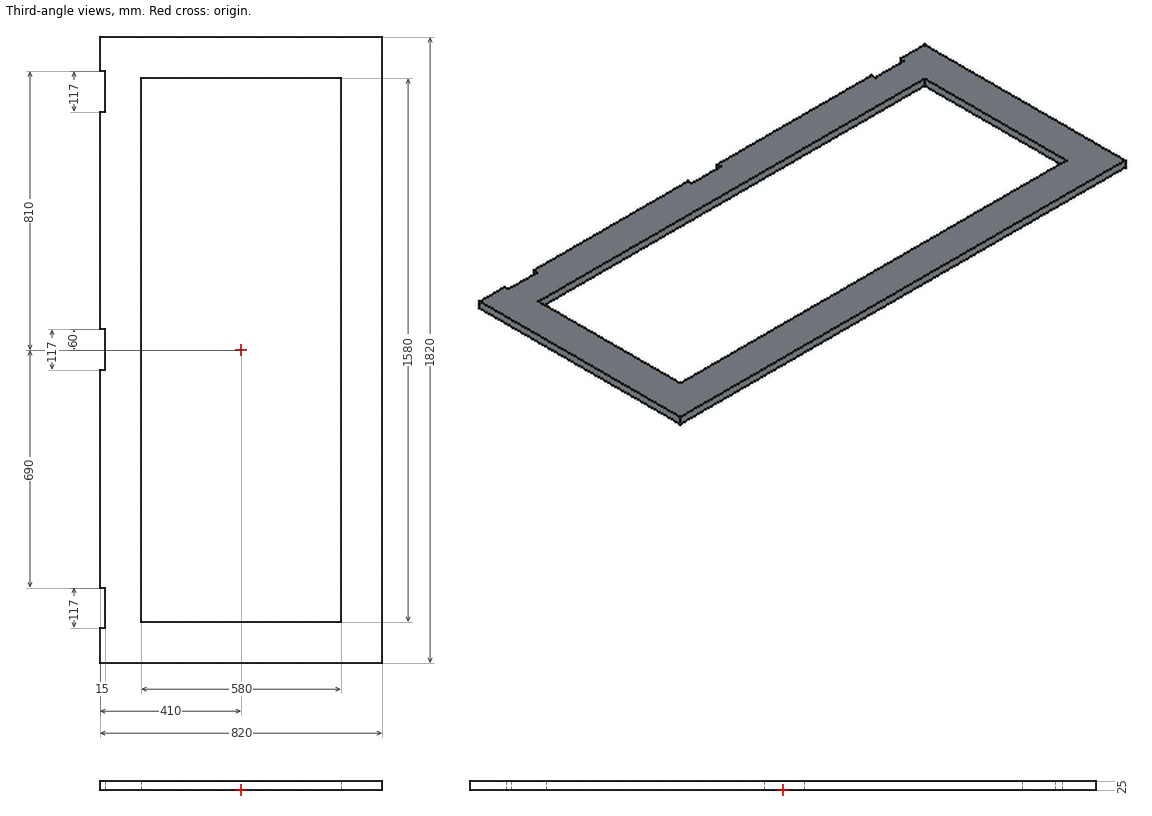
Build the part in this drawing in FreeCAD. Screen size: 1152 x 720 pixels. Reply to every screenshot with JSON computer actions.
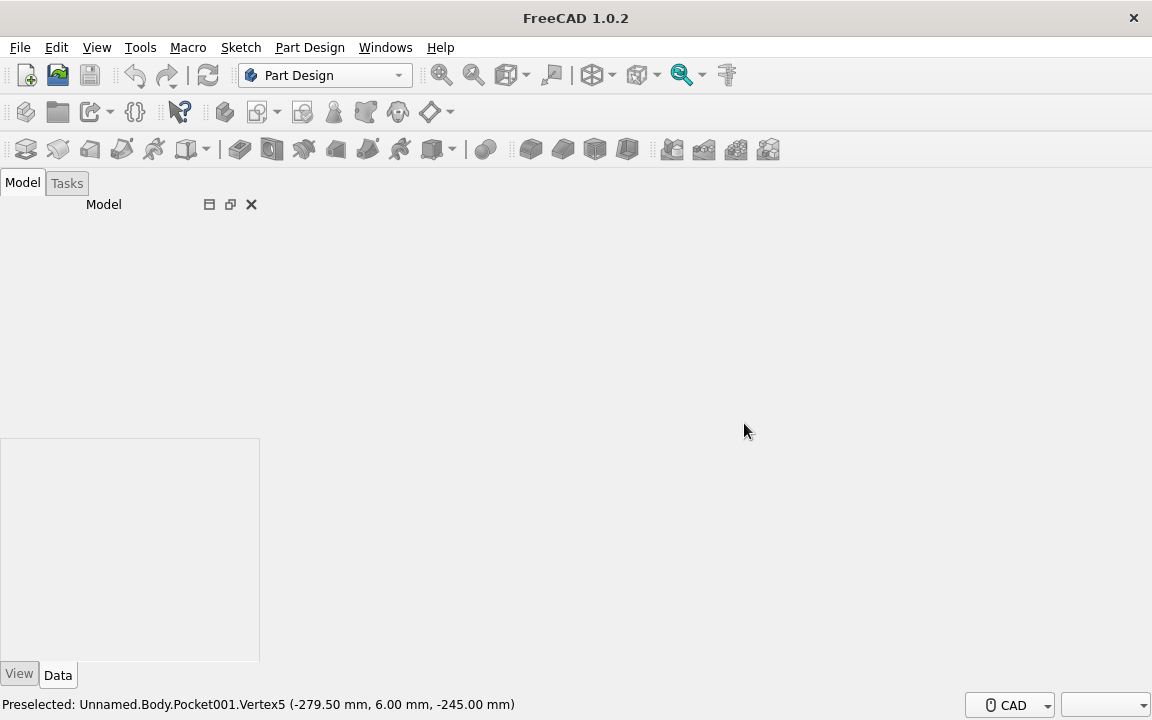
{"action": "left_click", "coordinate": [26, 76]}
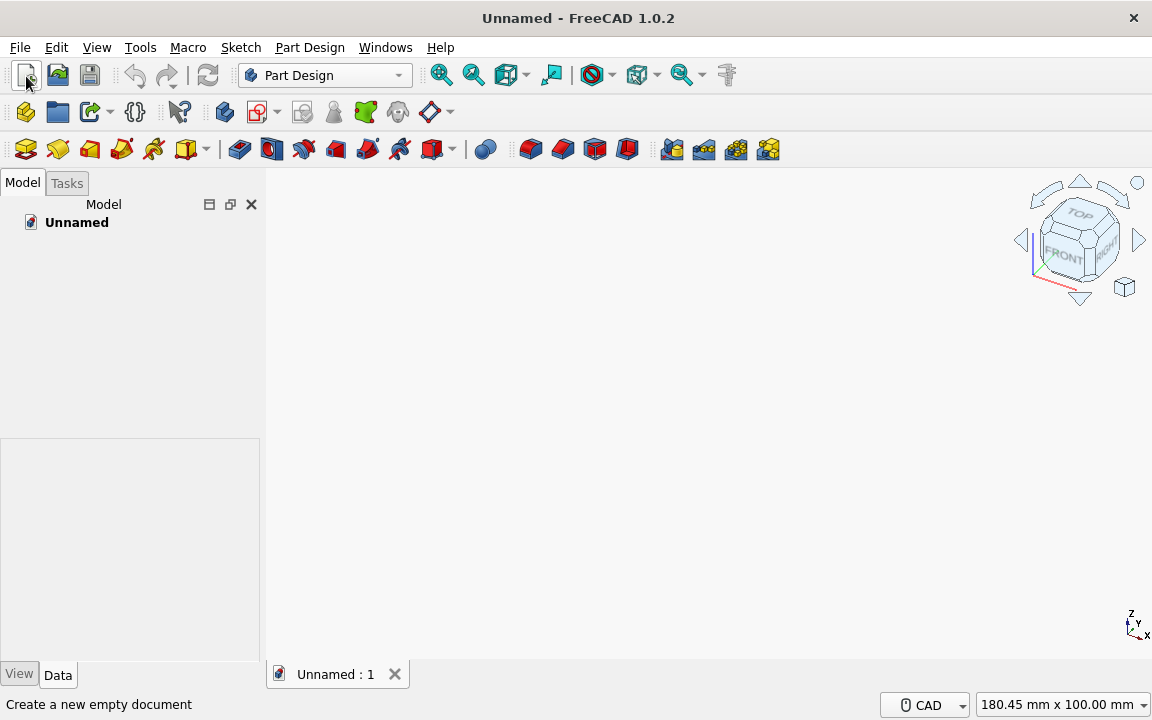
{"action": "left_click", "coordinate": [258, 112]}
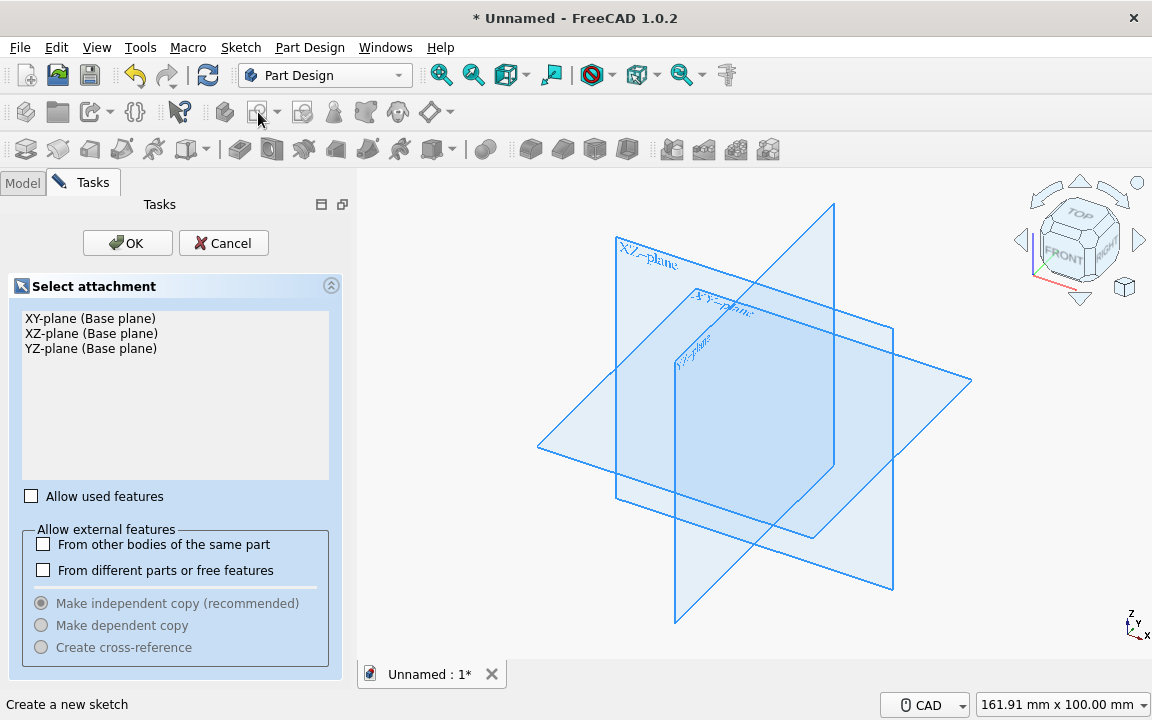
{"action": "left_click", "coordinate": [82, 318]}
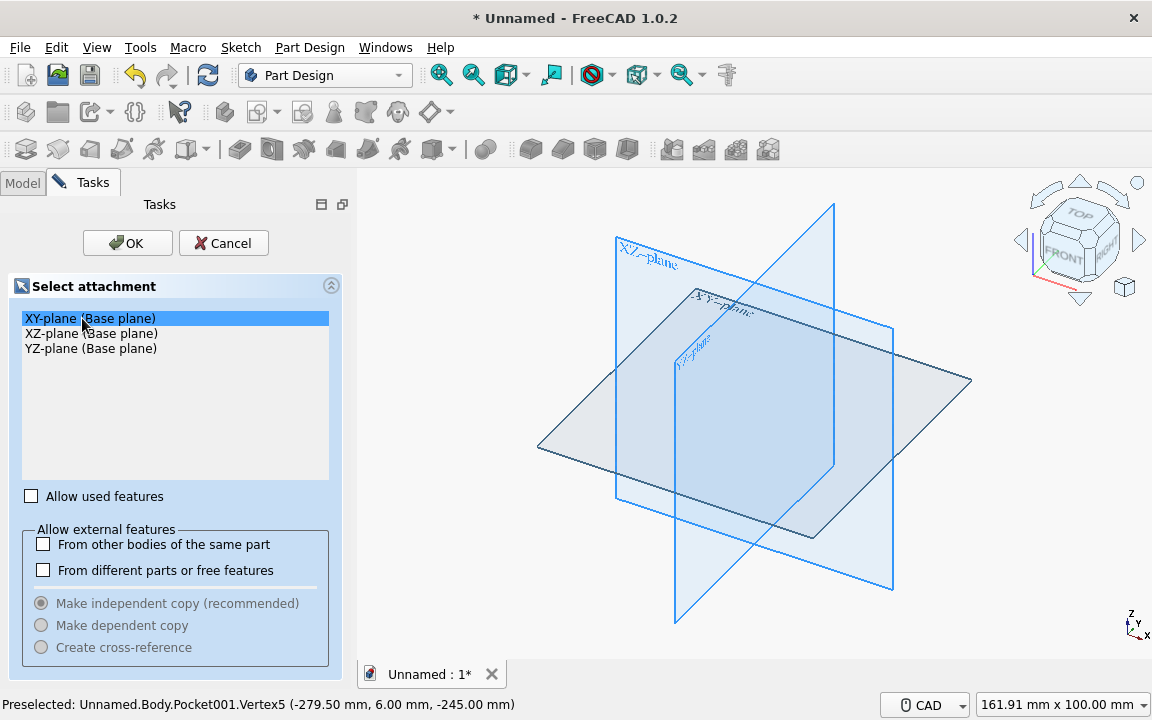
{"action": "left_click", "coordinate": [128, 243]}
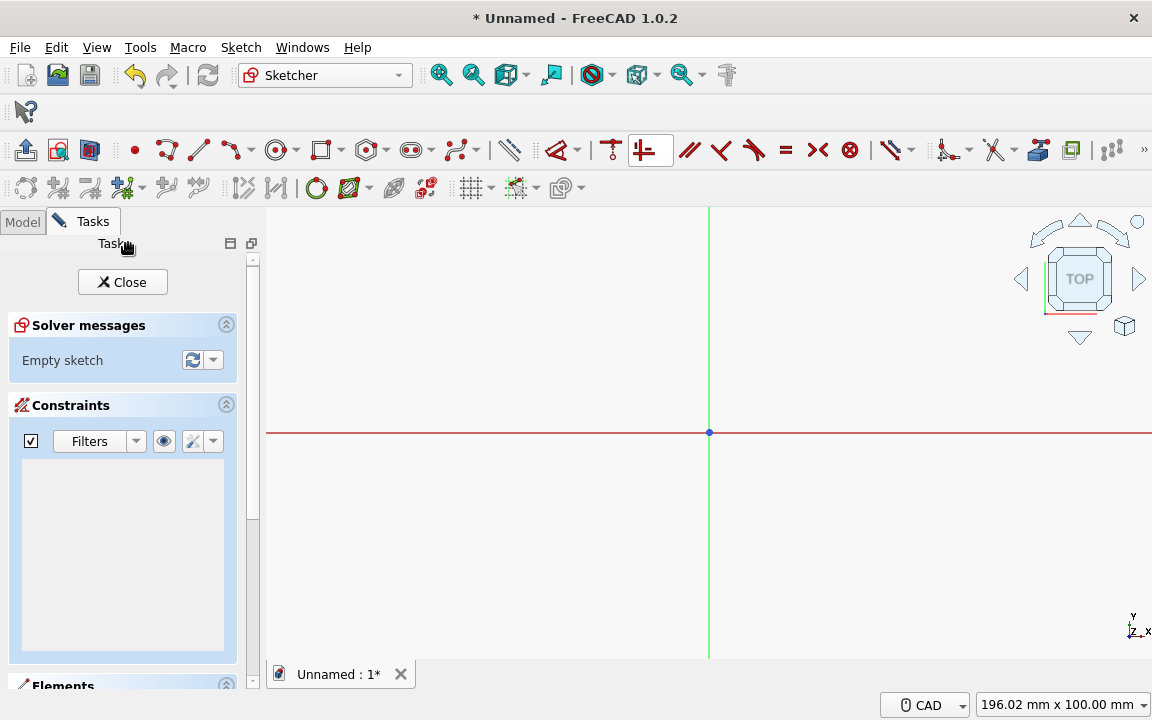
{"action": "scroll", "coordinate": [638, 433], "scroll_direction": "down", "scroll_amount": 16}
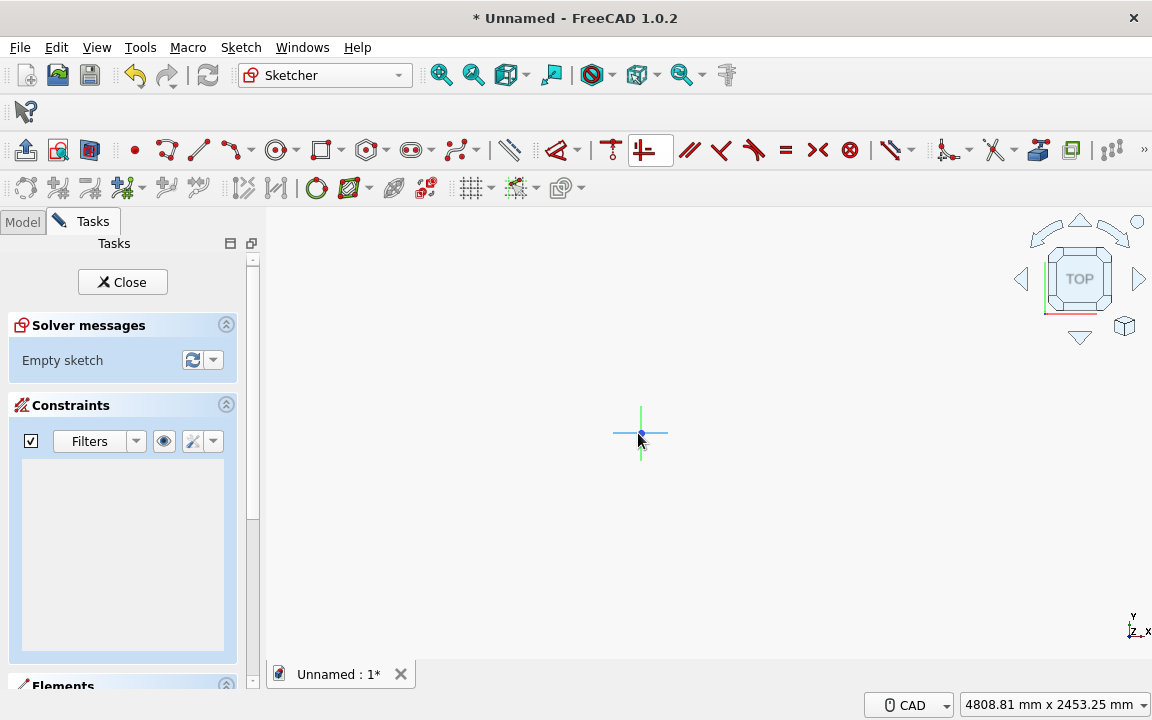
{"action": "left_click", "coordinate": [344, 150]}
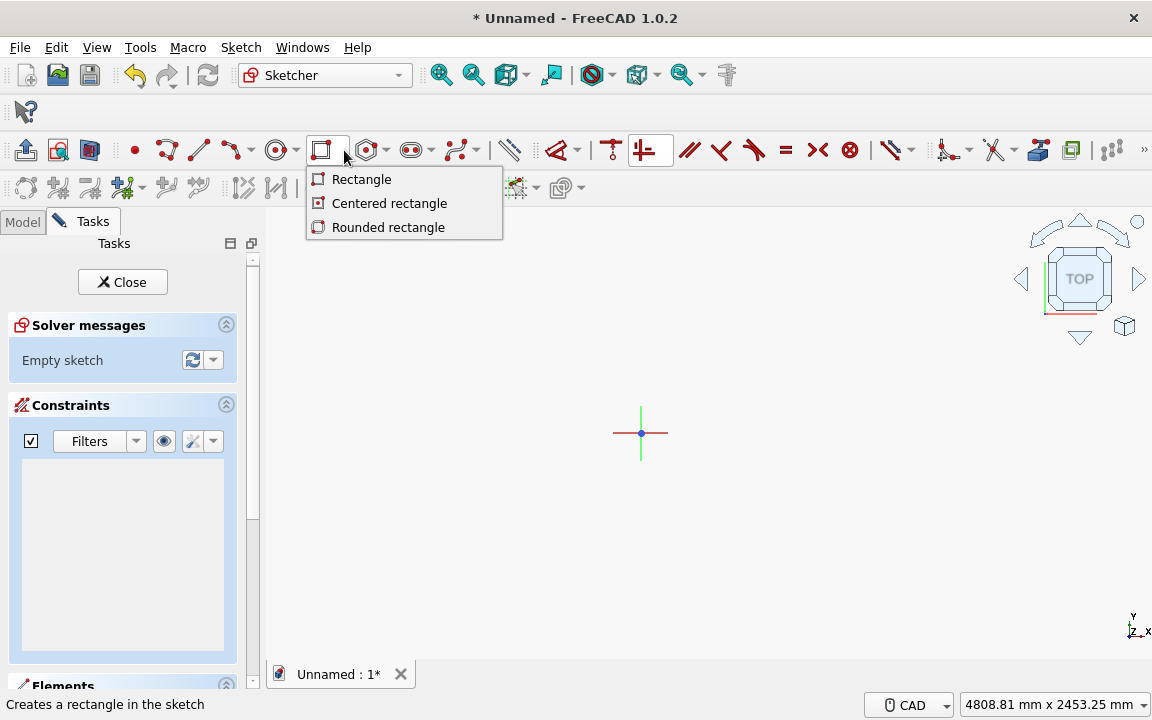
{"action": "left_click", "coordinate": [404, 203]}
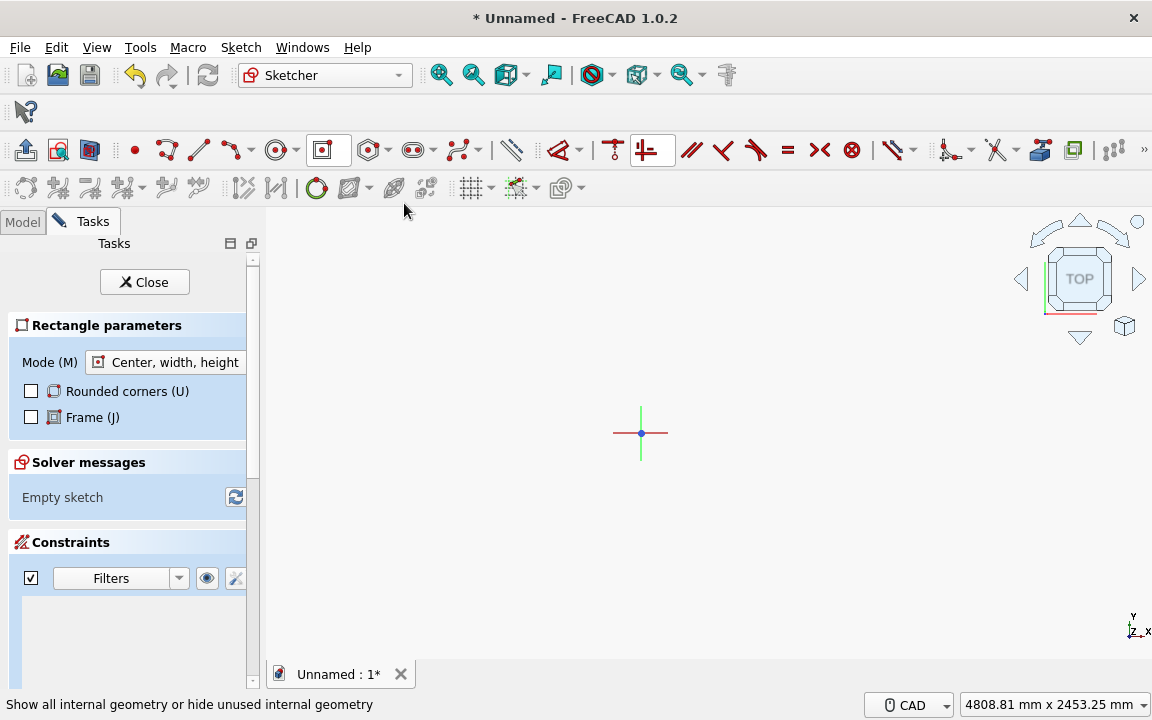
{"action": "left_click", "coordinate": [641, 433]}
{"action": "mouse_move", "coordinate": [717, 266]}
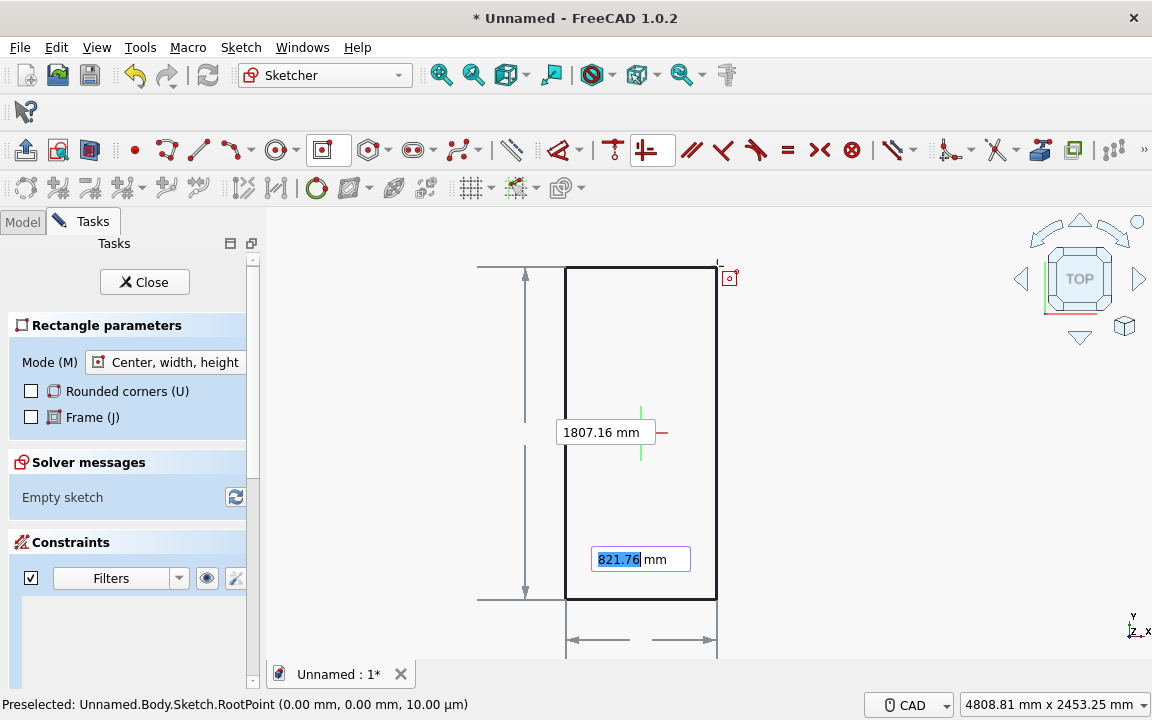
{"action": "type", "text": "820"}
{"action": "key", "text": "Tab"}
{"action": "type", "text": "1820"}
{"action": "key", "text": "Return"}
{"action": "key", "text": "Escape"}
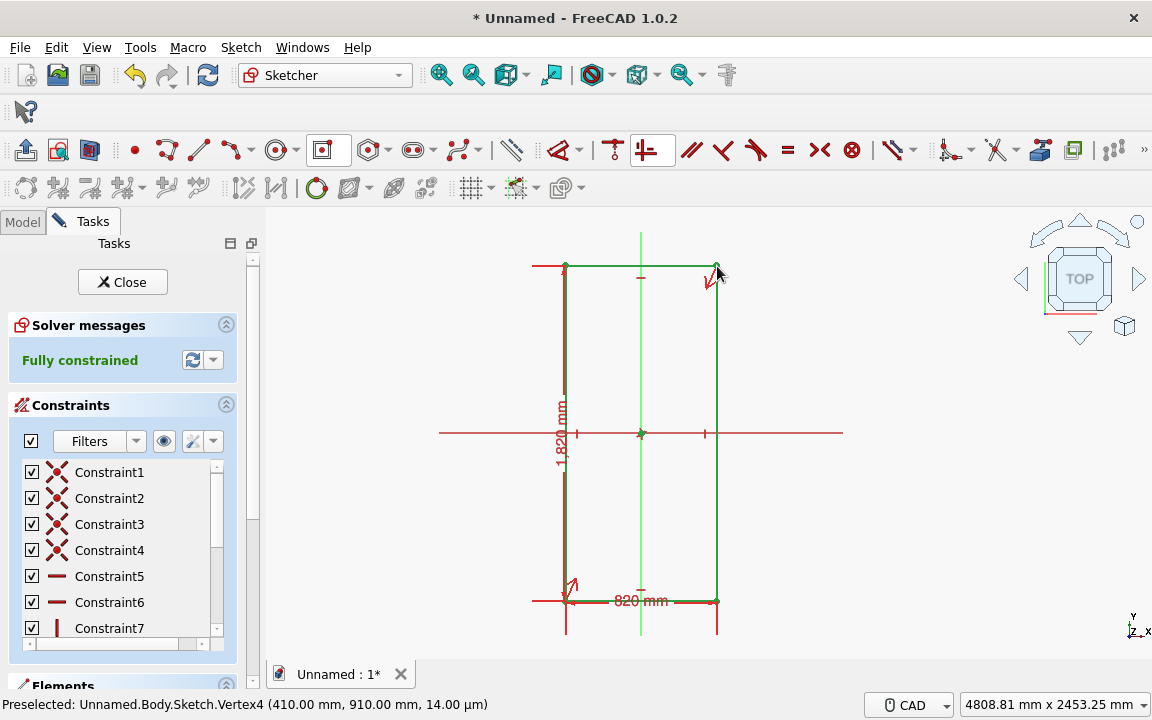
{"action": "left_click", "coordinate": [123, 282]}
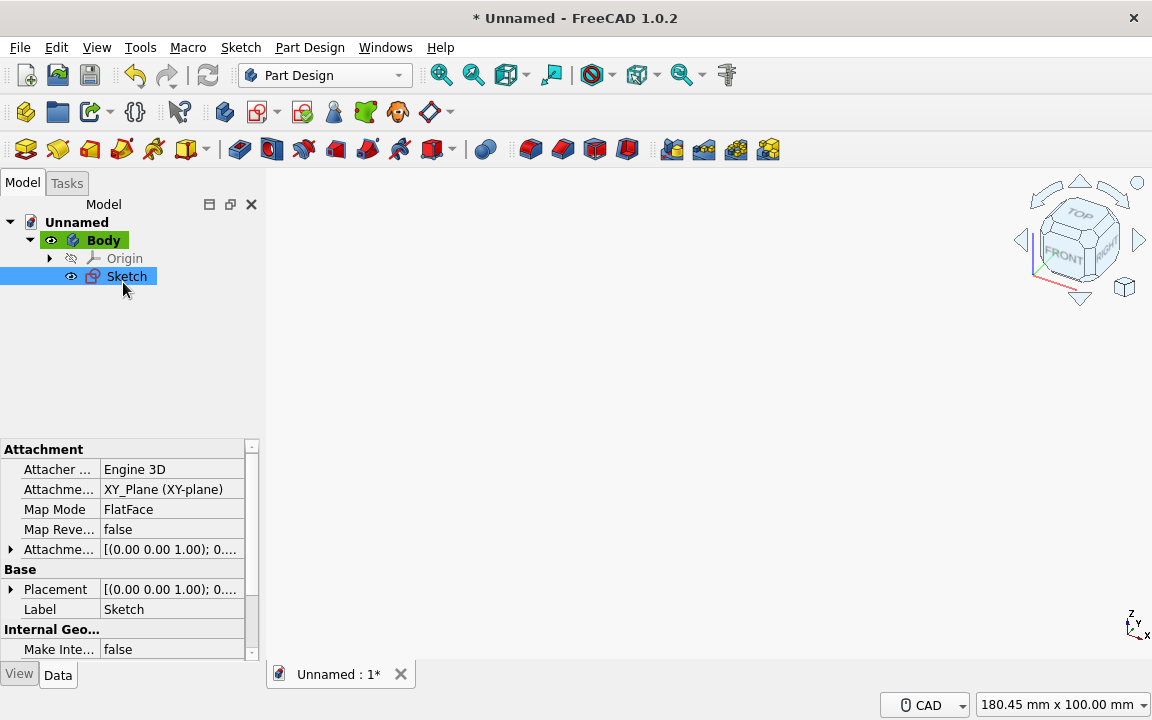
{"action": "left_click", "coordinate": [26, 150]}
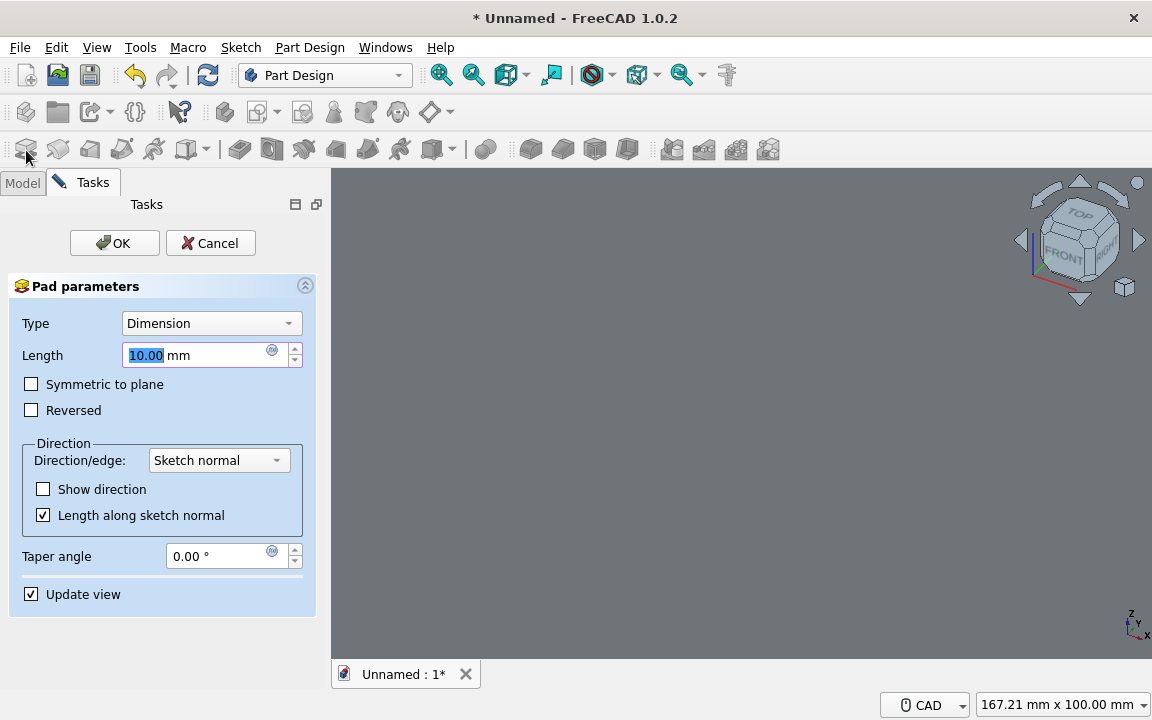
{"action": "type", "text": "25"}
{"action": "key", "text": "Tab"}